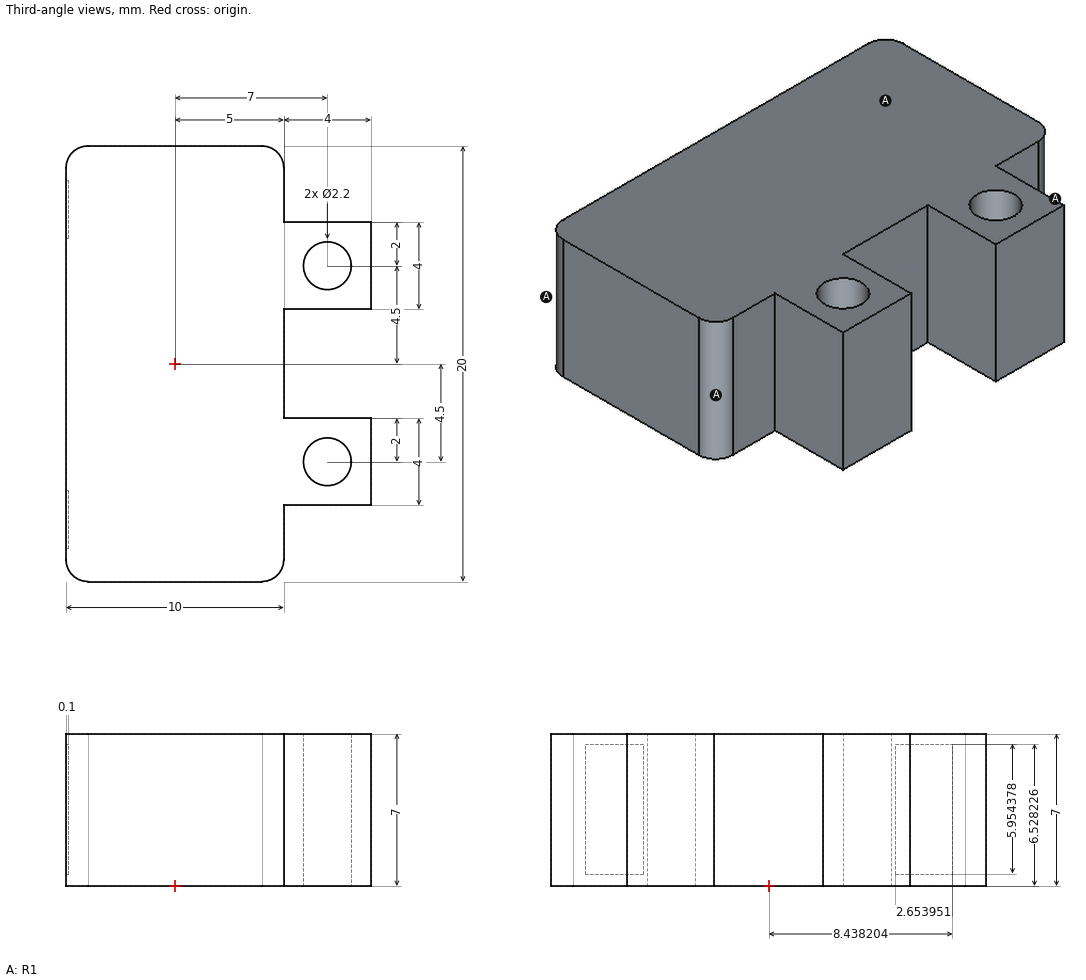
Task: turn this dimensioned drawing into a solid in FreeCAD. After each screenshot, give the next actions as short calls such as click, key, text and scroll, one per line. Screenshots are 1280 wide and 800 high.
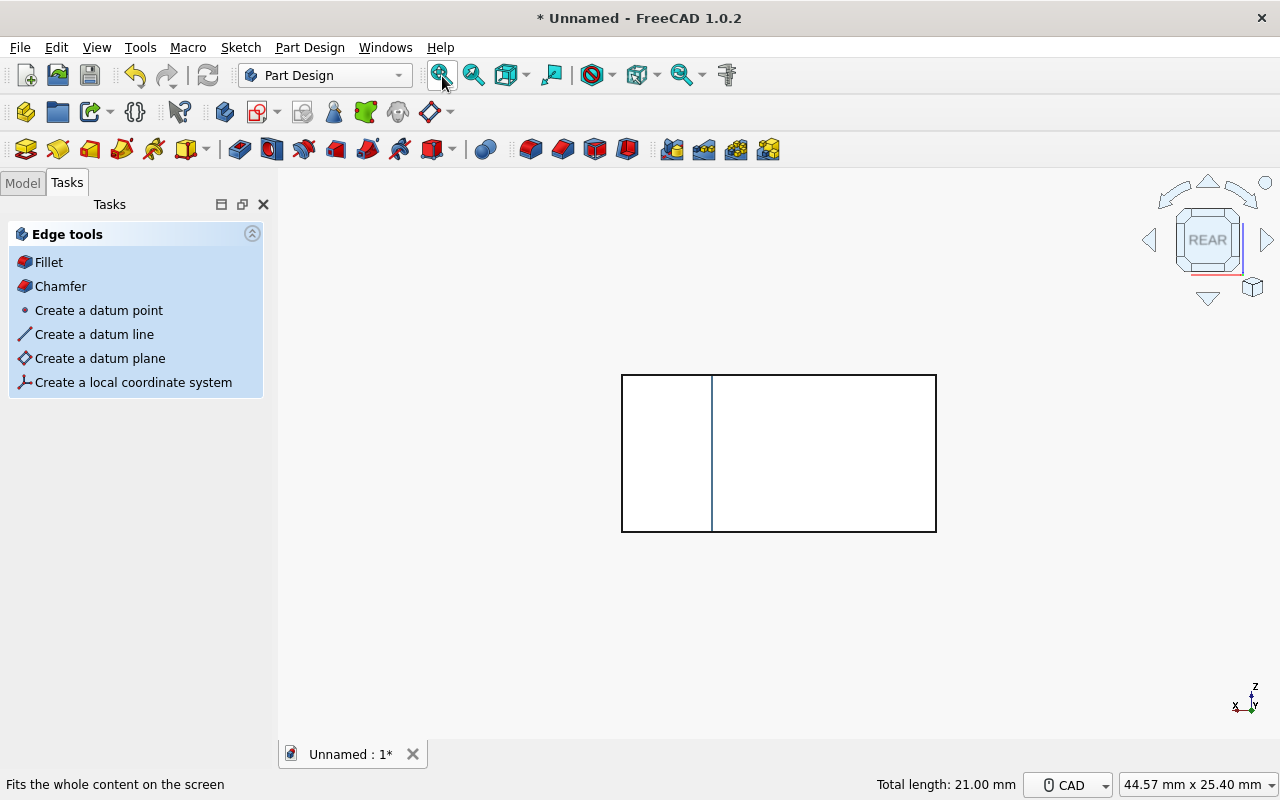
click(936, 453, ctrl)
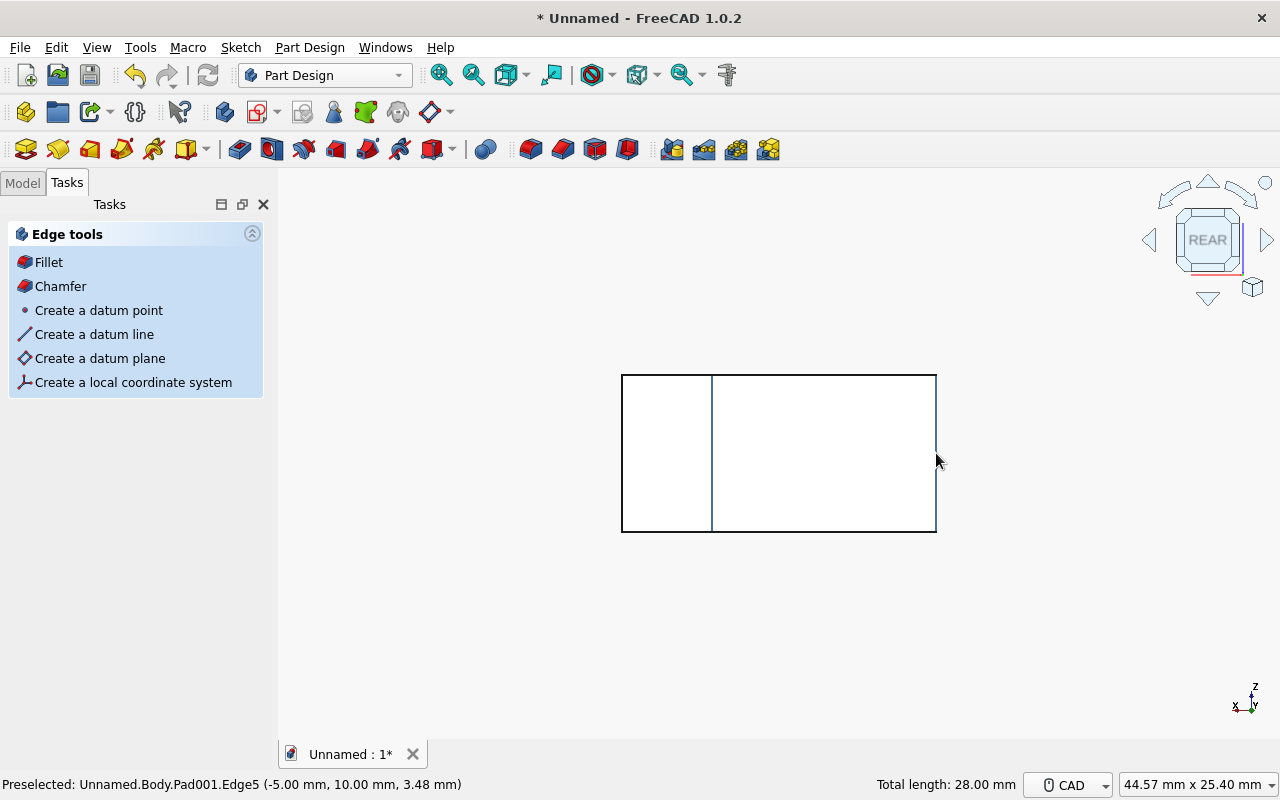
click(532, 150)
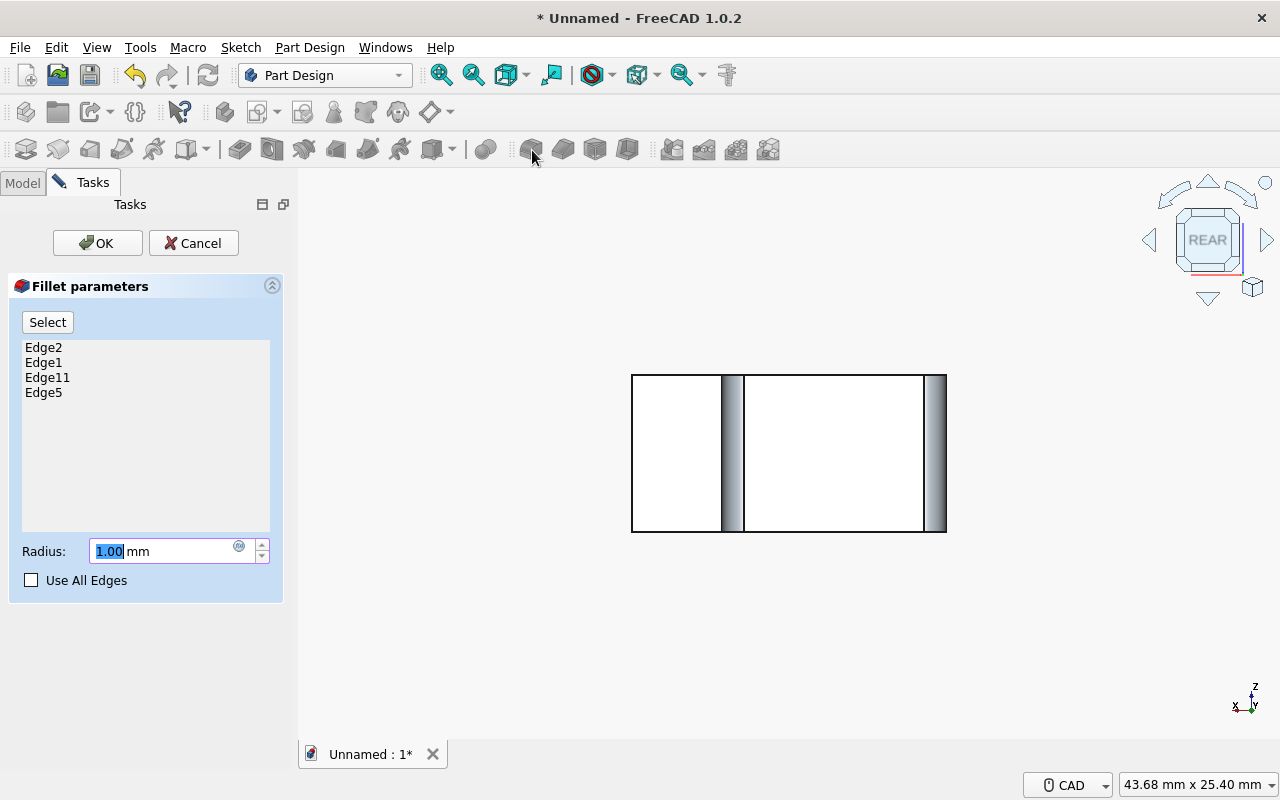
text(1)
key(Tab)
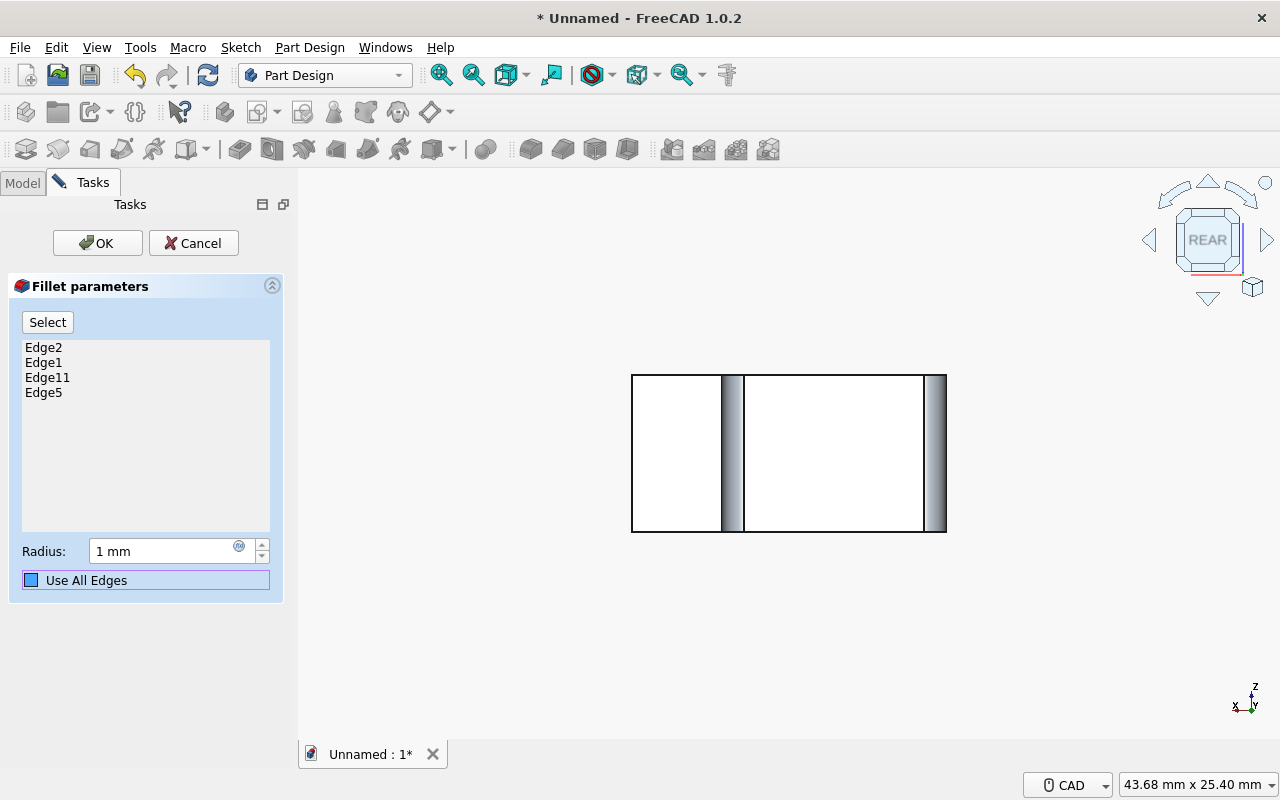
click(98, 243)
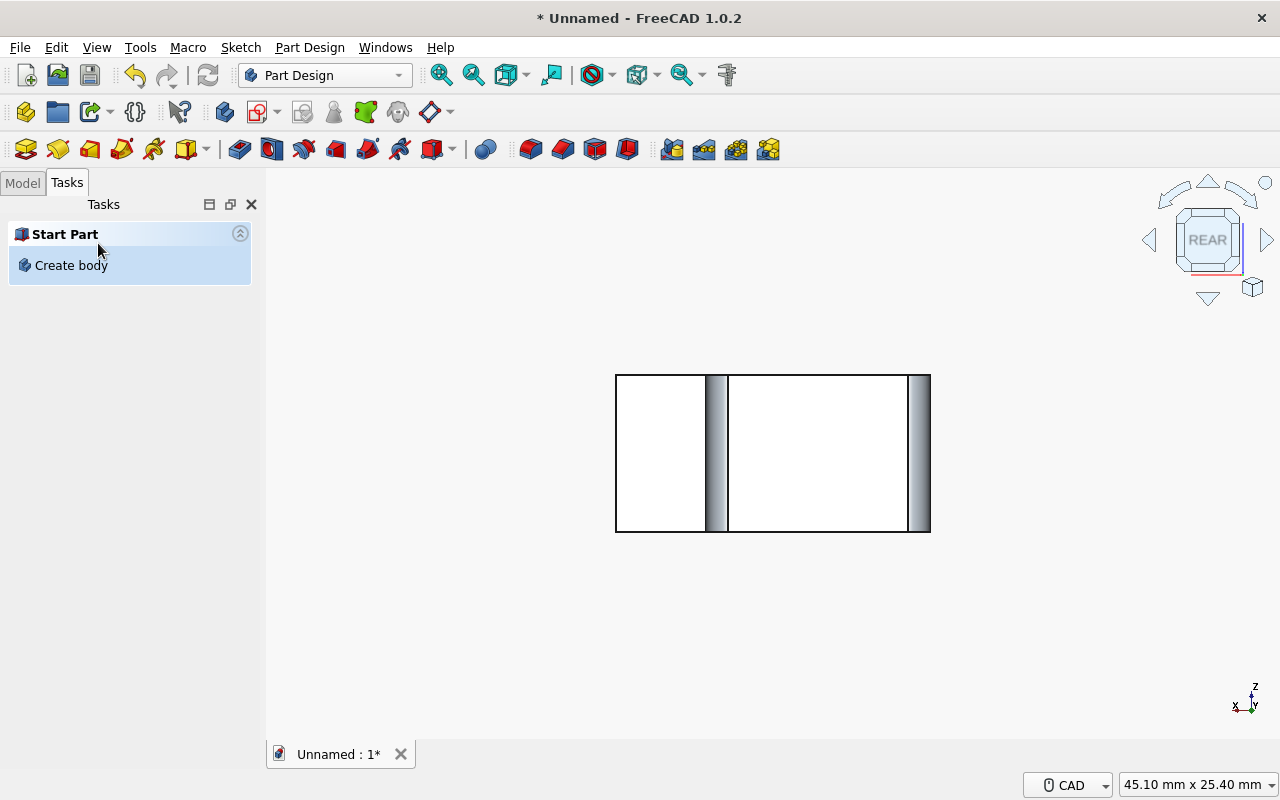
key(v)
key(f)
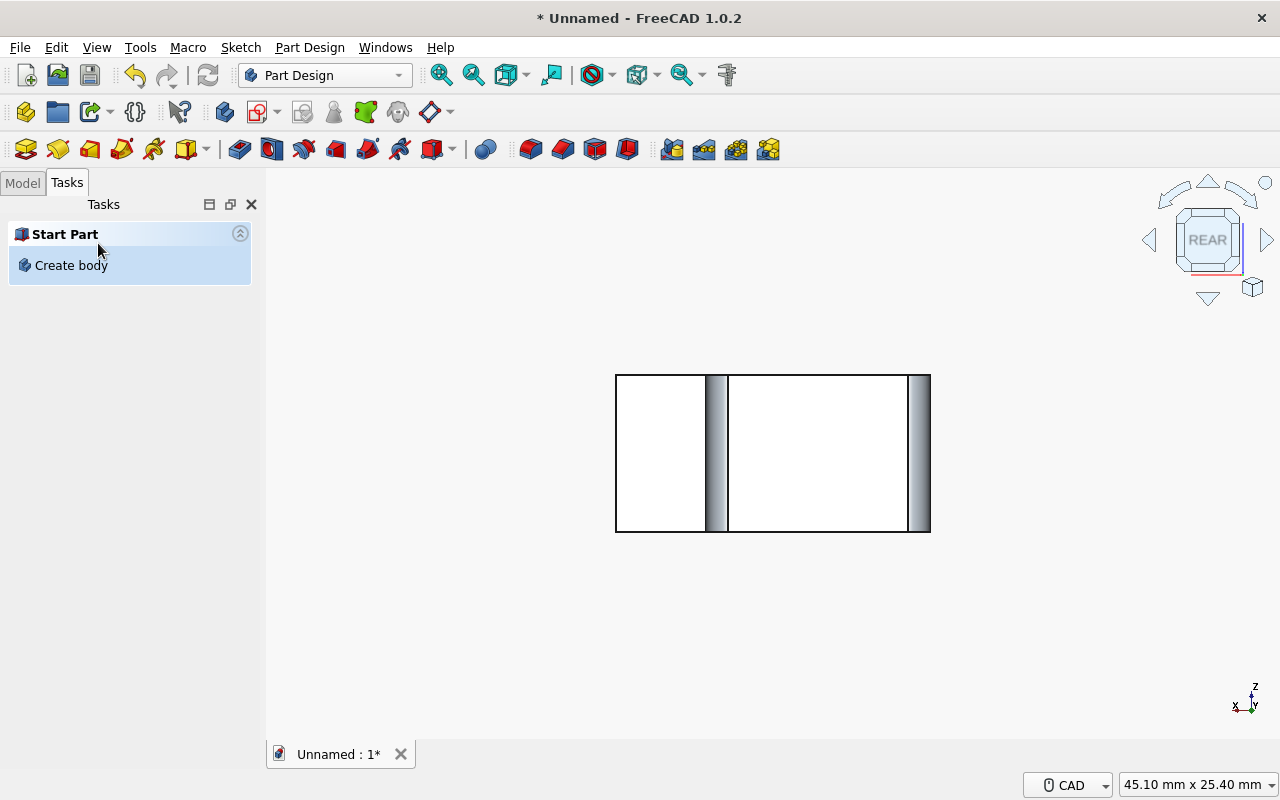
key(6)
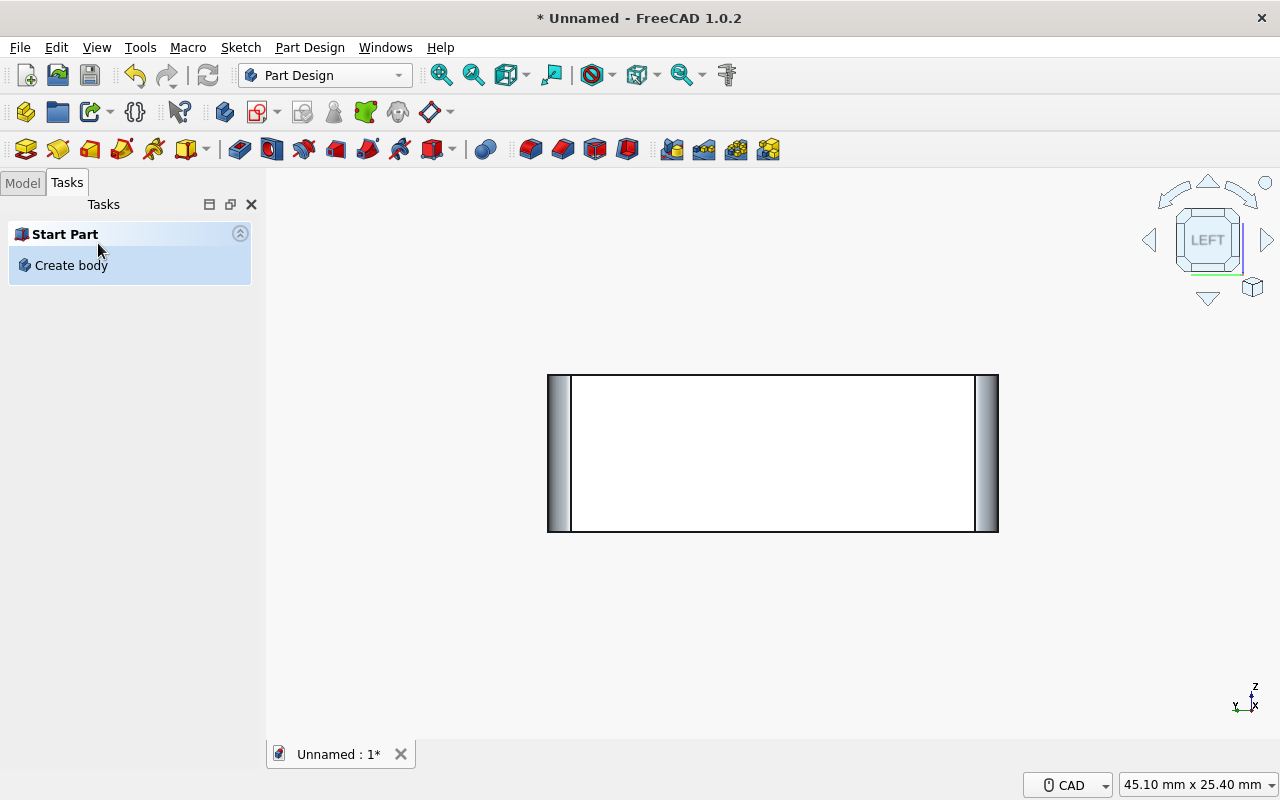
key(v)
key(f)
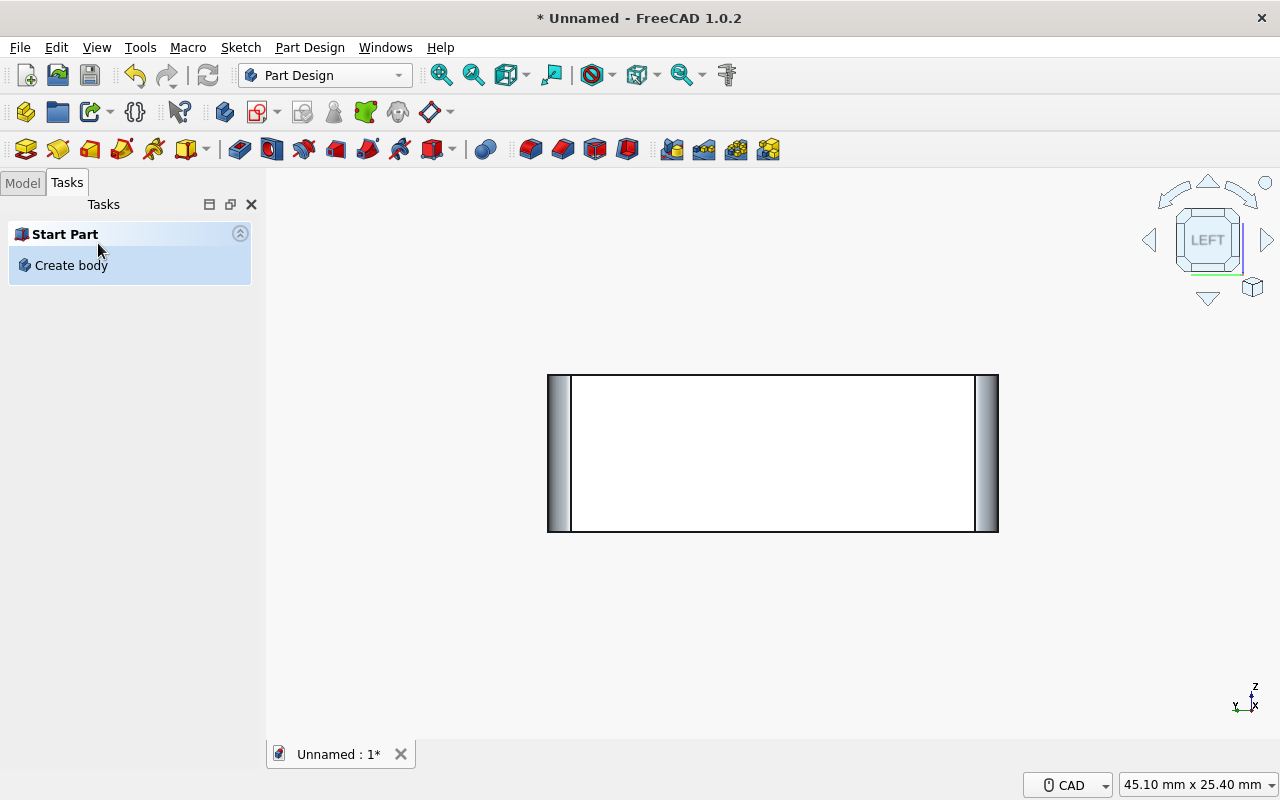
click(657, 452)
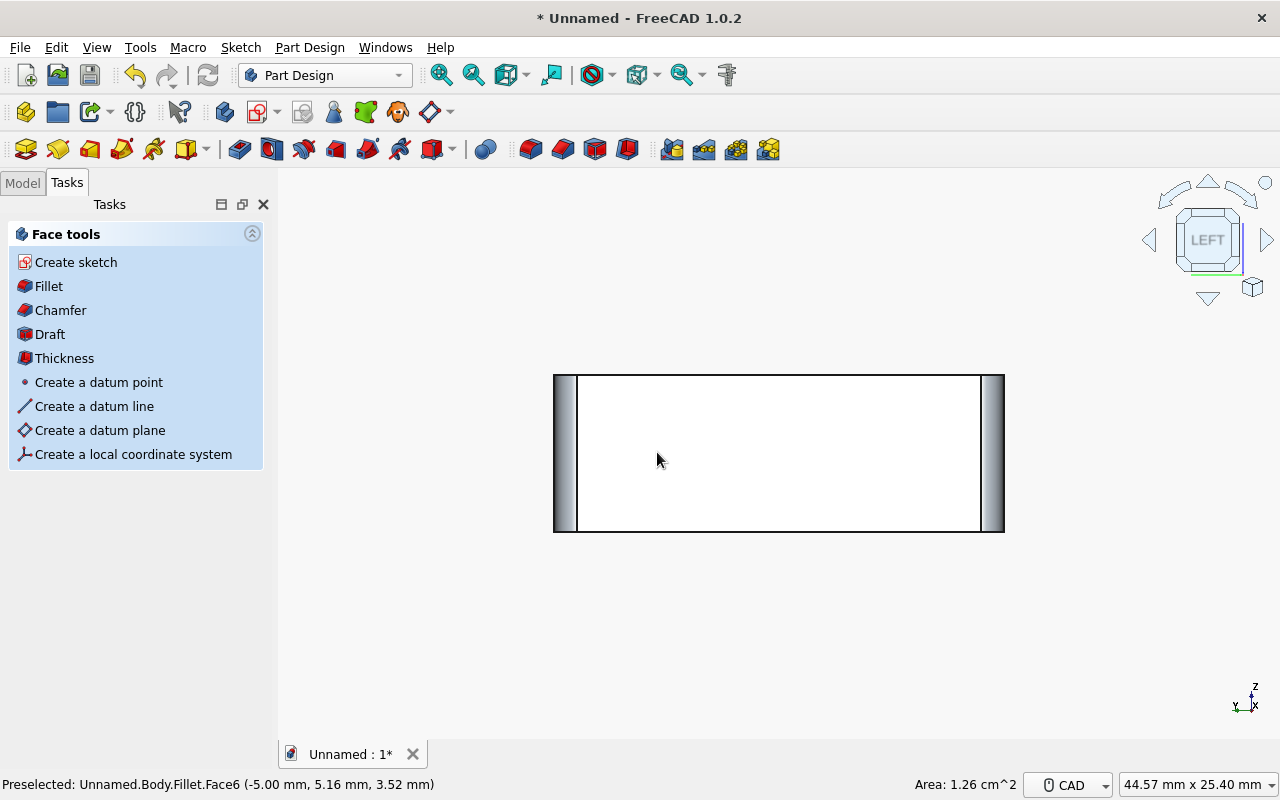
click(258, 112)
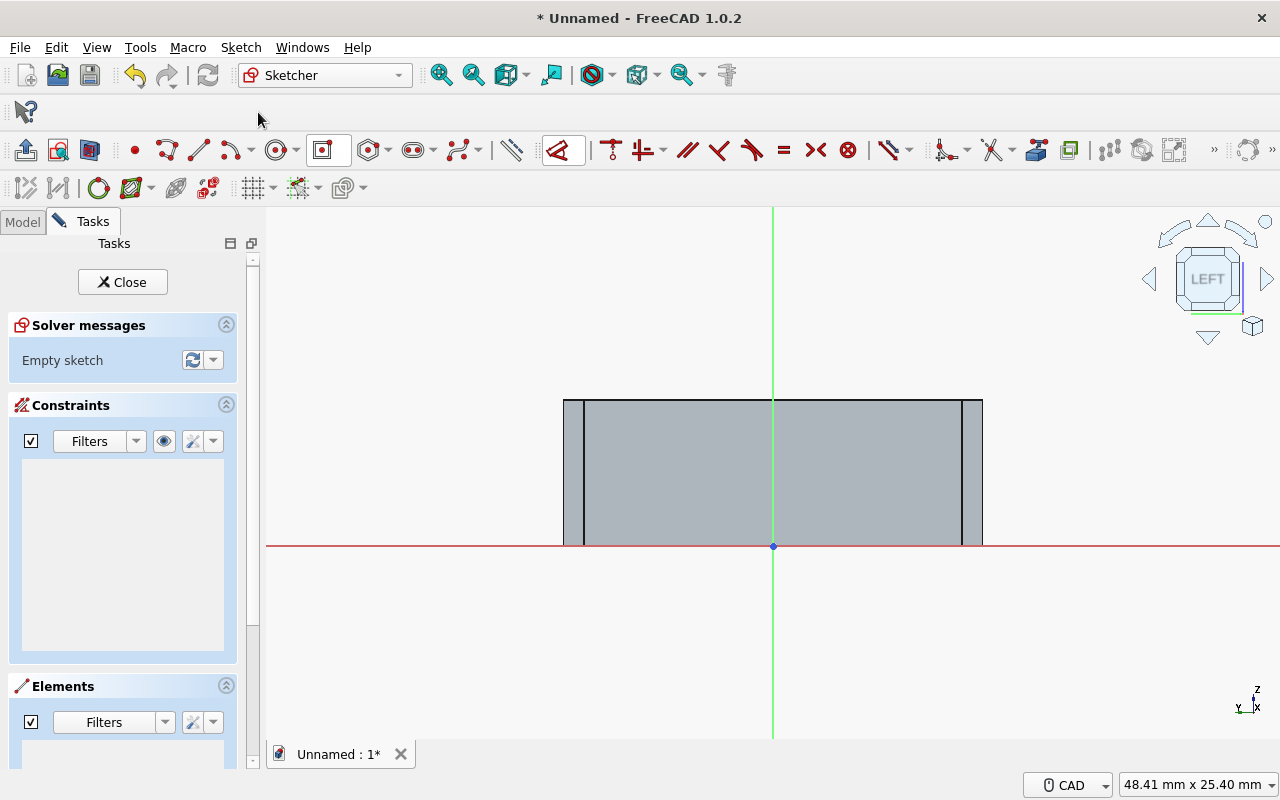
scroll(668, 482, up, 4)